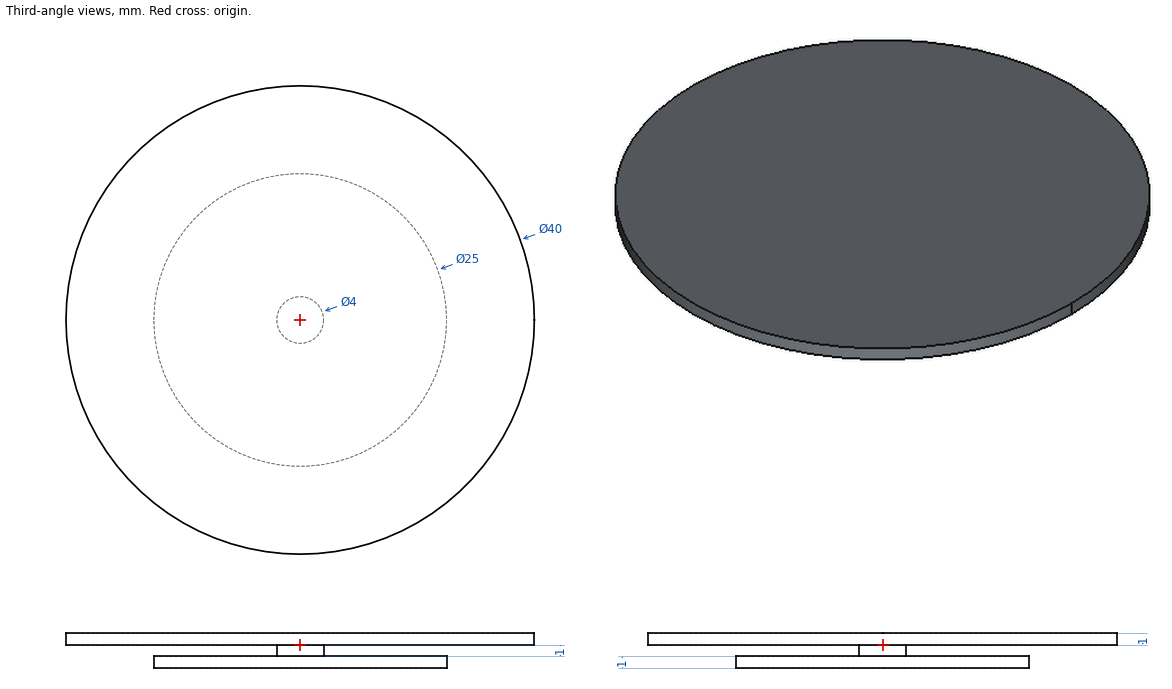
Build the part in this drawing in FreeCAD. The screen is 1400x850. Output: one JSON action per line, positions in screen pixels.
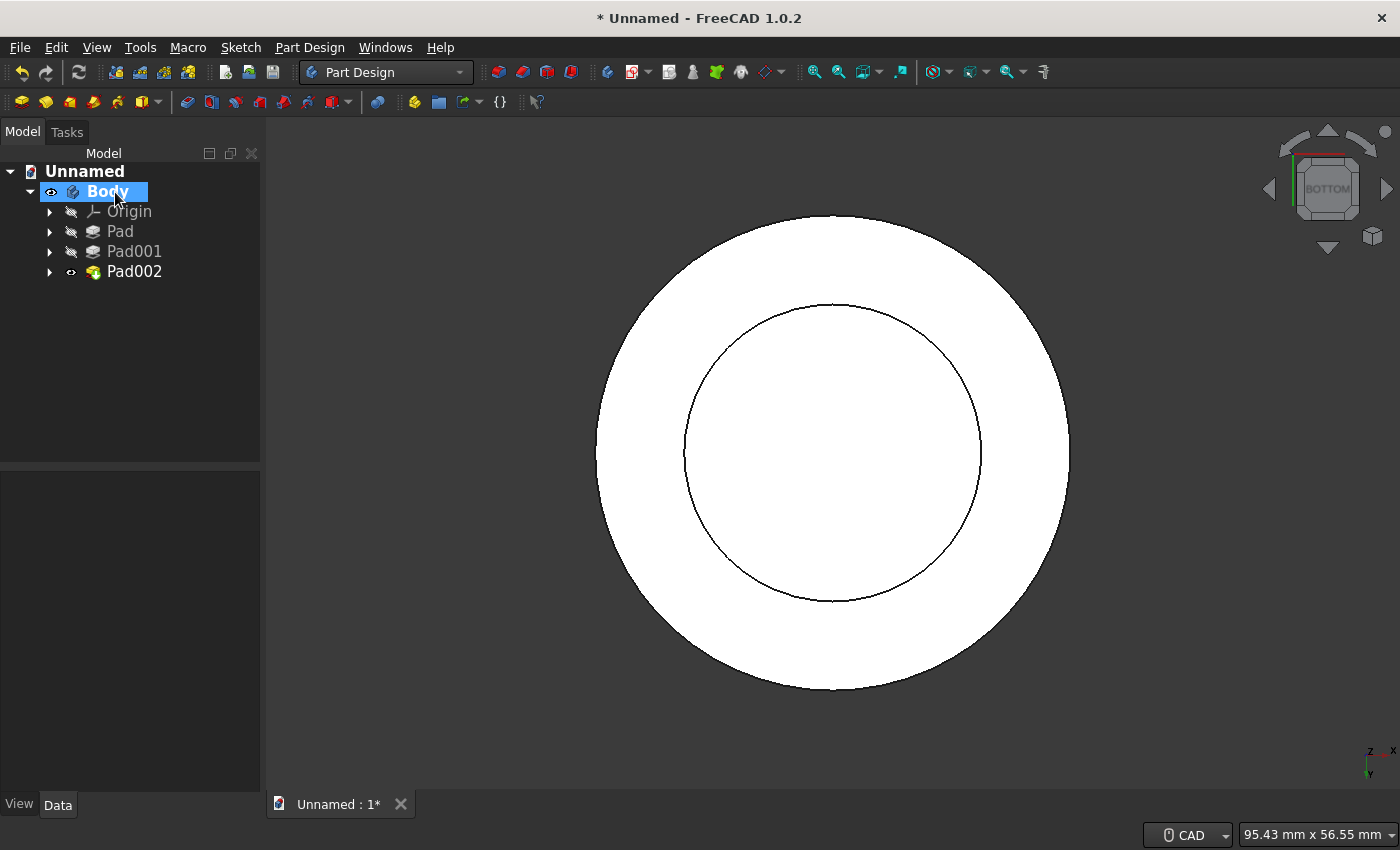
{"action": "key", "text": "0"}